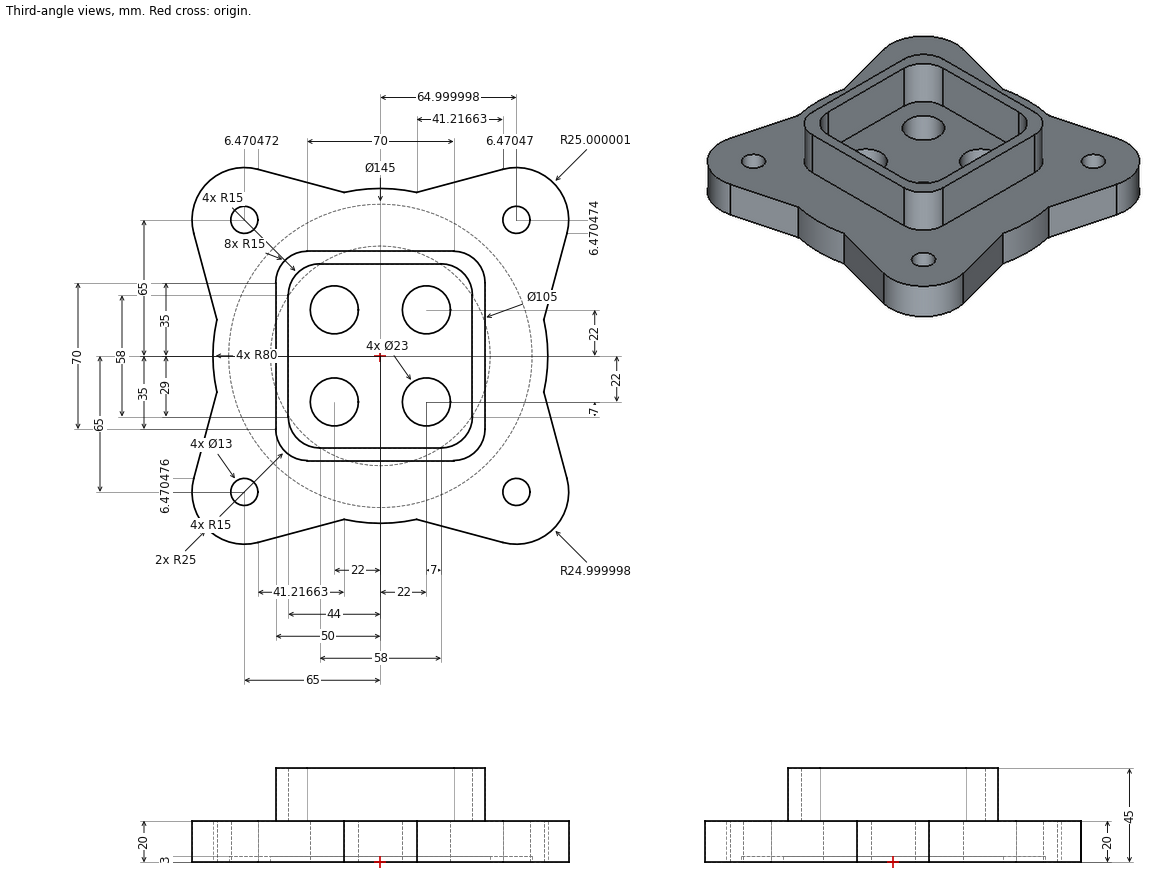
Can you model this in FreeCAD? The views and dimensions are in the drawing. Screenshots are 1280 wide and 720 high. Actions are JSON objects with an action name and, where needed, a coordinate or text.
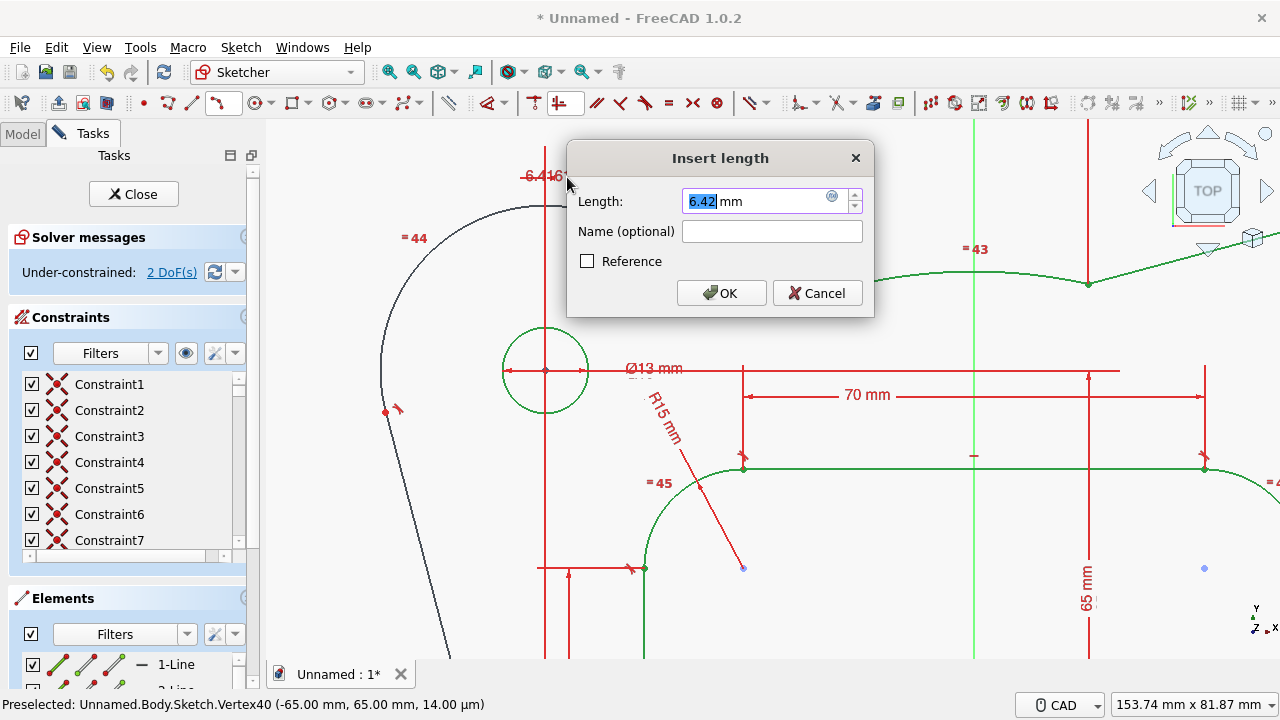
{"action": "type", "text": "6.470472"}
{"action": "key", "text": "Return"}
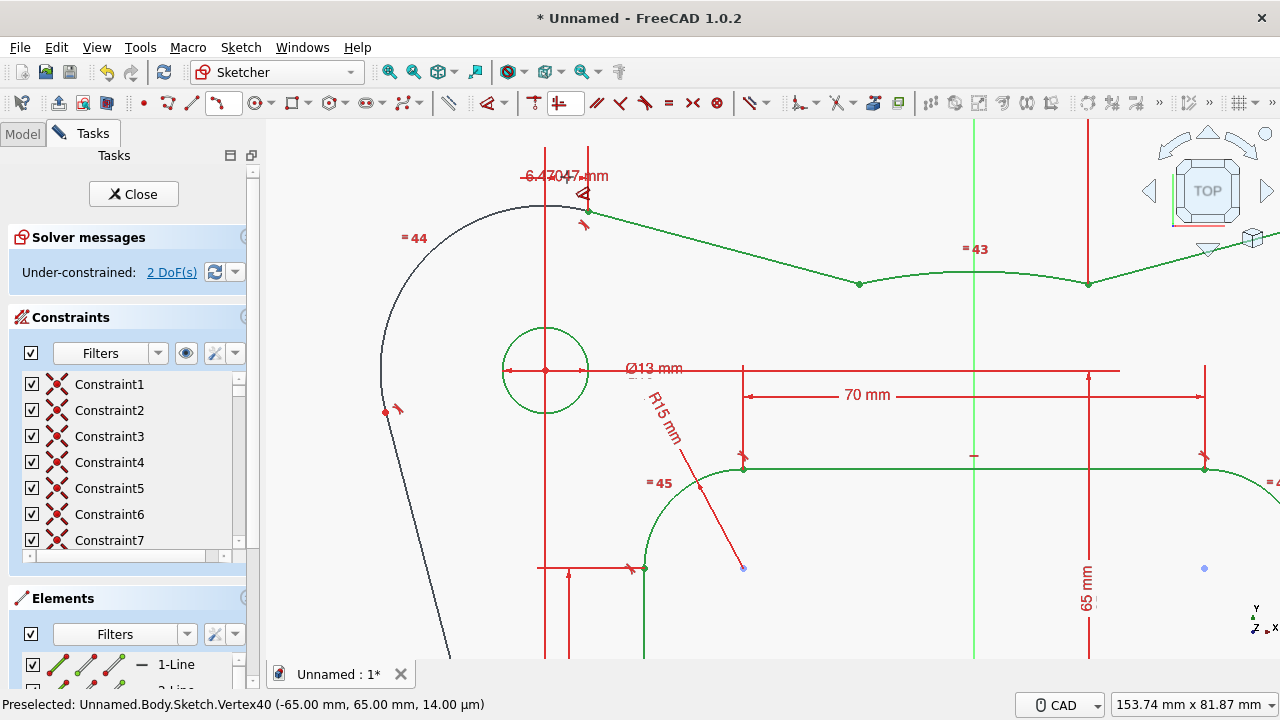
{"action": "left_click", "coordinate": [386, 412]}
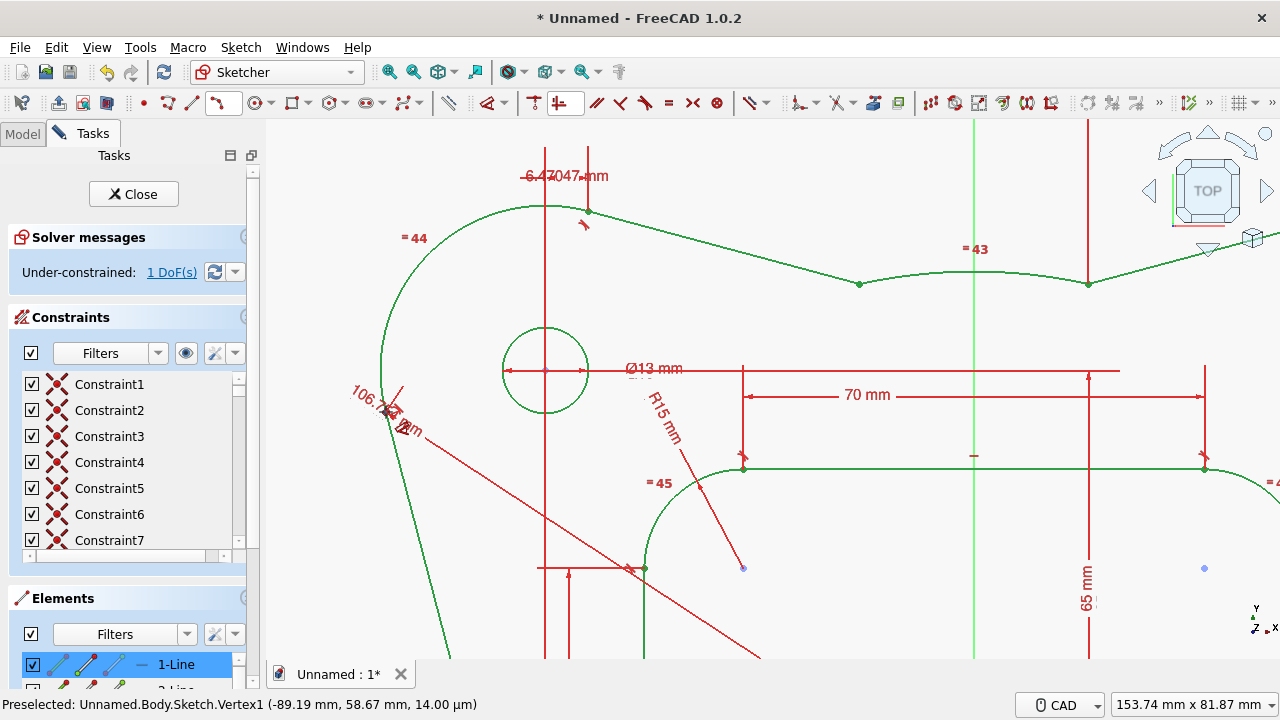
{"action": "left_click", "coordinate": [545, 371]}
{"action": "left_click", "coordinate": [352, 391]}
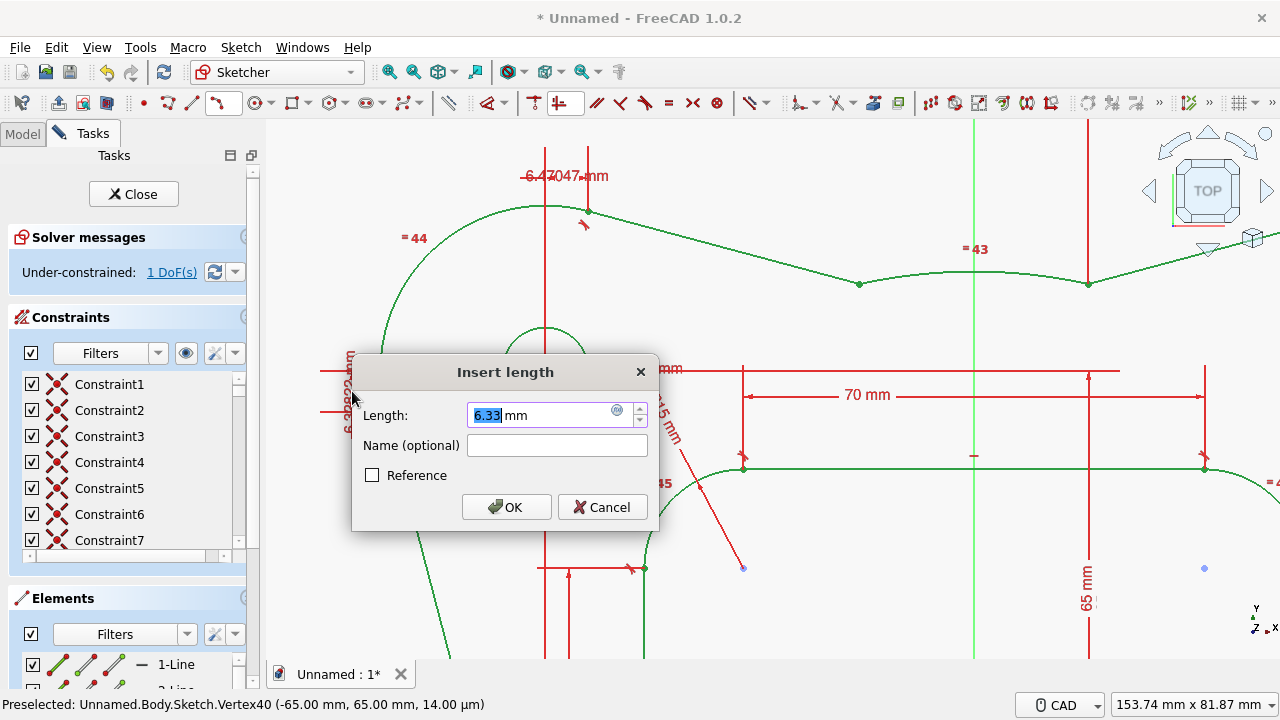
{"action": "type", "text": "6.470476"}
{"action": "key", "text": "Return"}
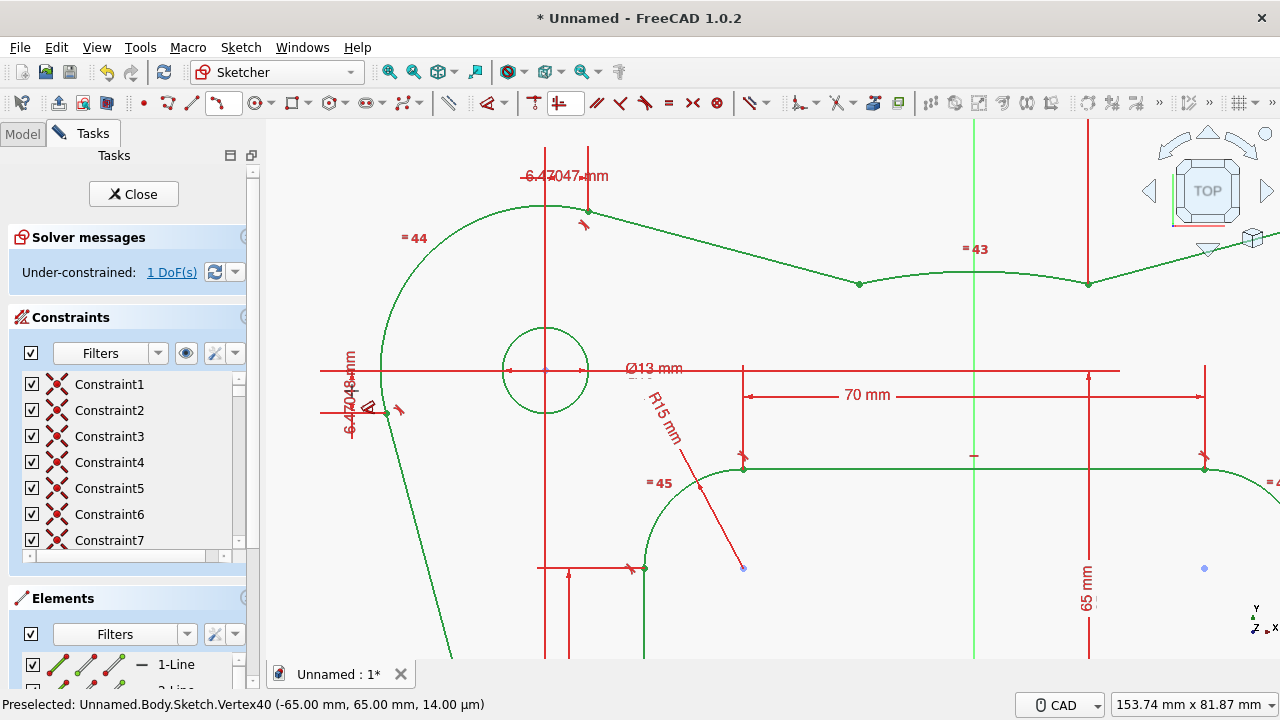
{"action": "scroll", "coordinate": [588, 212], "scroll_direction": "down", "scroll_amount": 6}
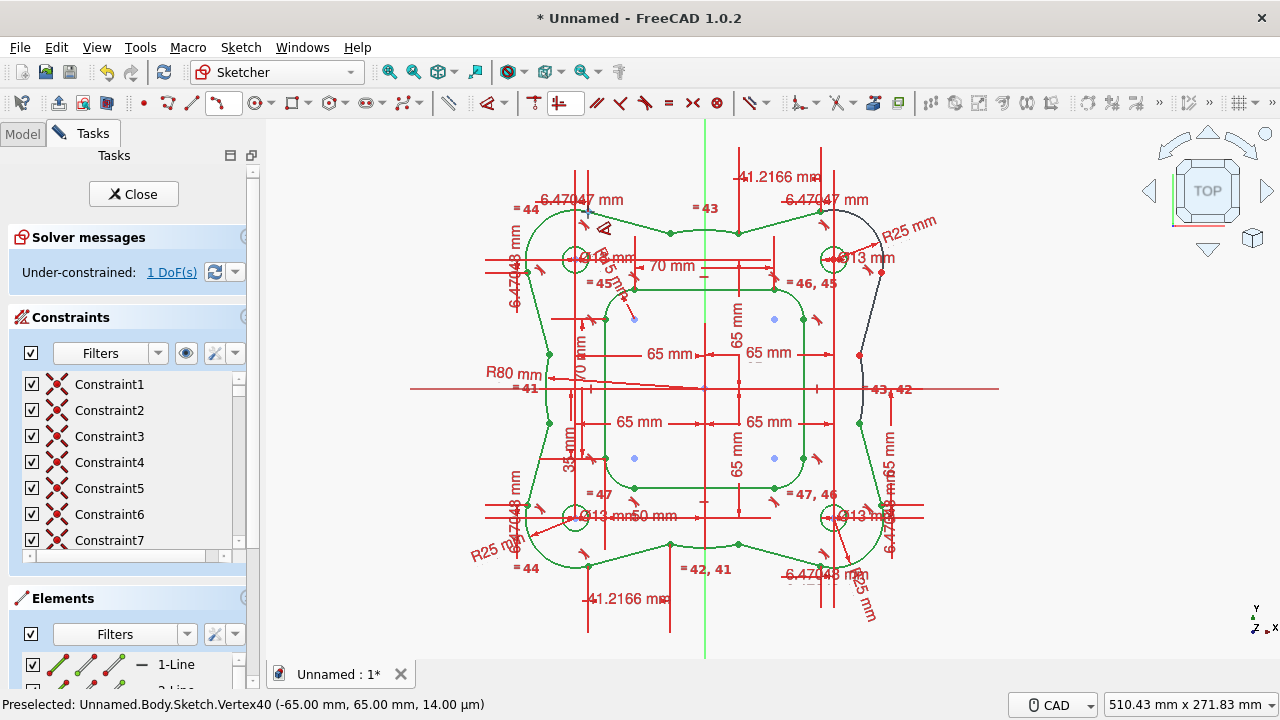
{"action": "scroll", "coordinate": [882, 272], "scroll_direction": "up", "scroll_amount": 6}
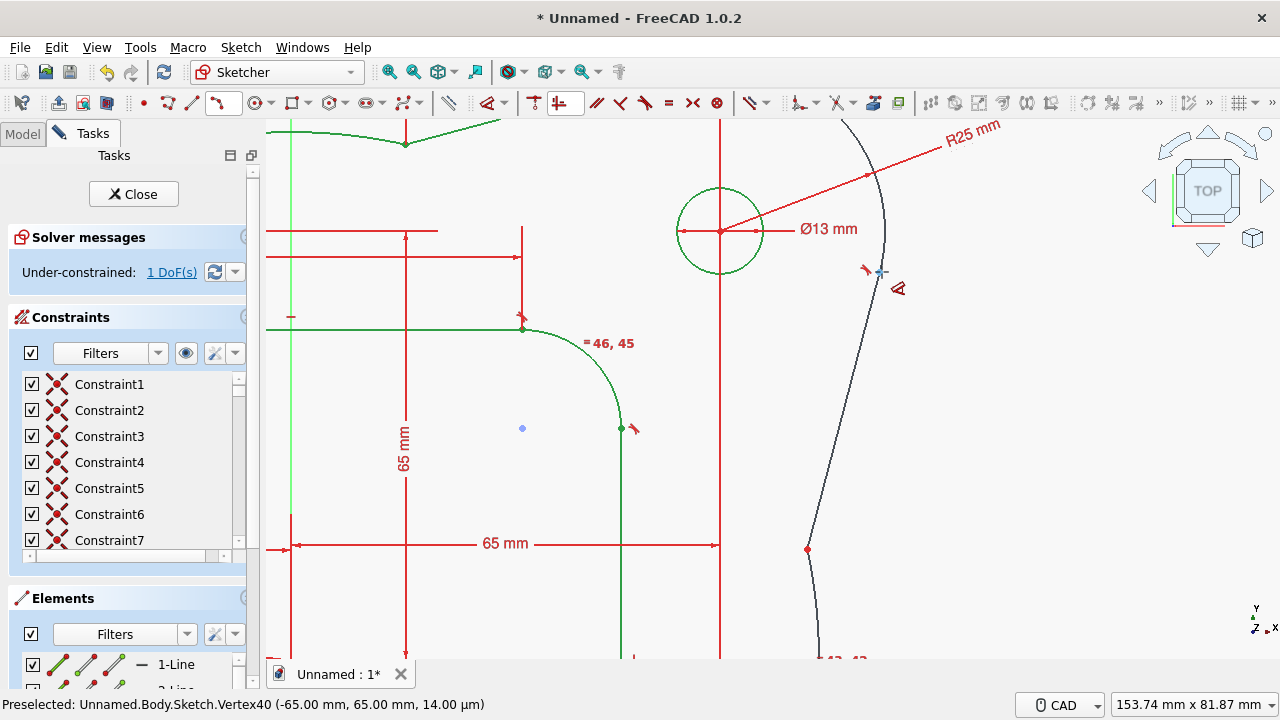
{"action": "left_click", "coordinate": [880, 273]}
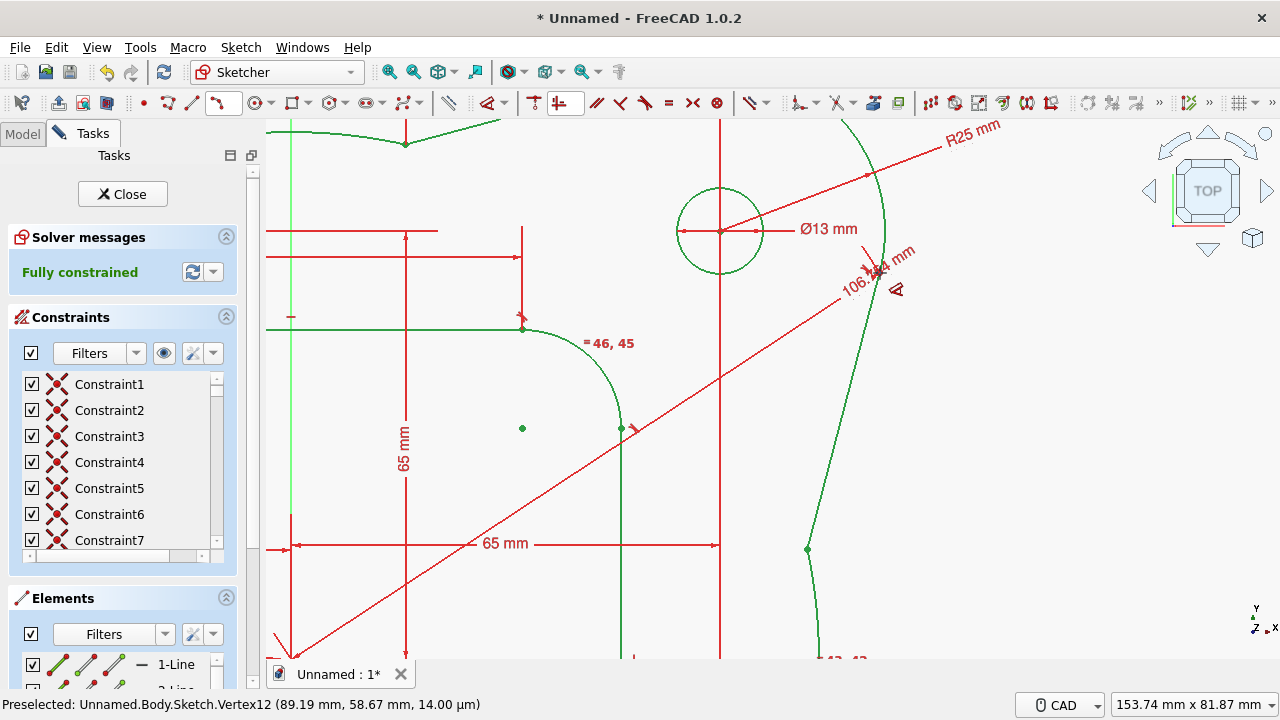
{"action": "left_click", "coordinate": [720, 231]}
{"action": "left_click", "coordinate": [914, 252]}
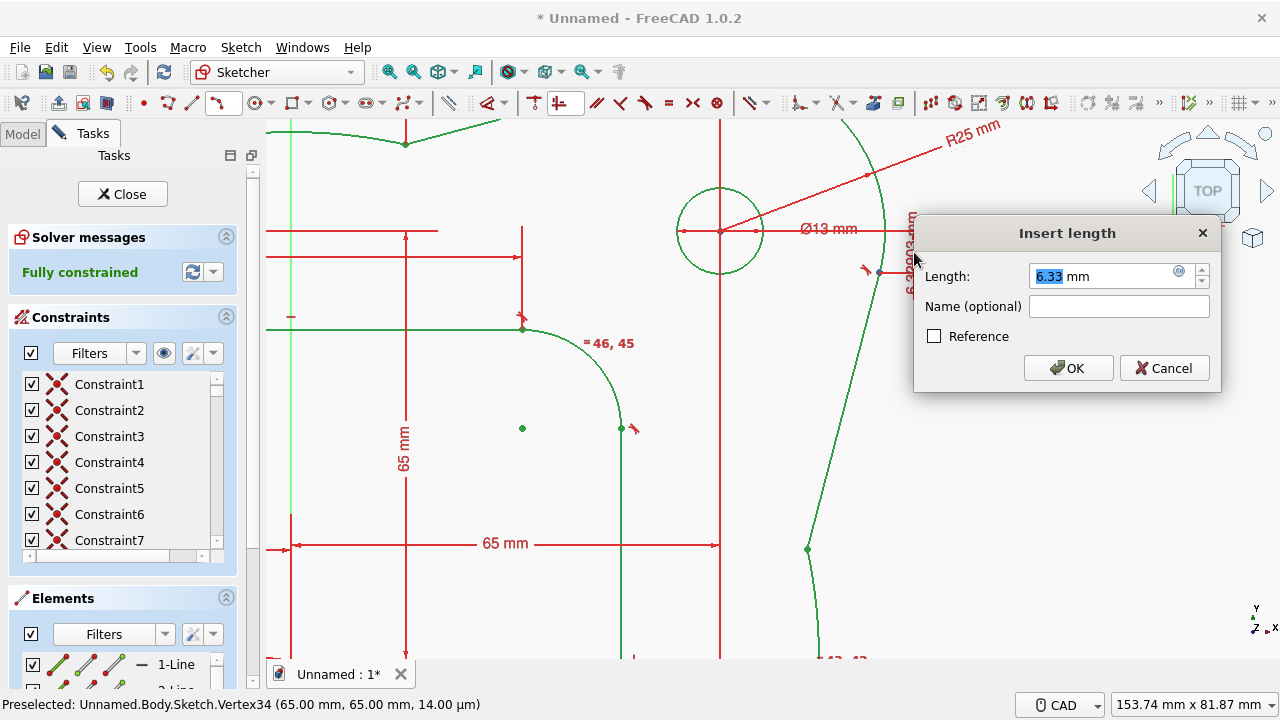
{"action": "type", "text": "6.470474"}
{"action": "key", "text": "Return"}
{"action": "key", "text": "Escape"}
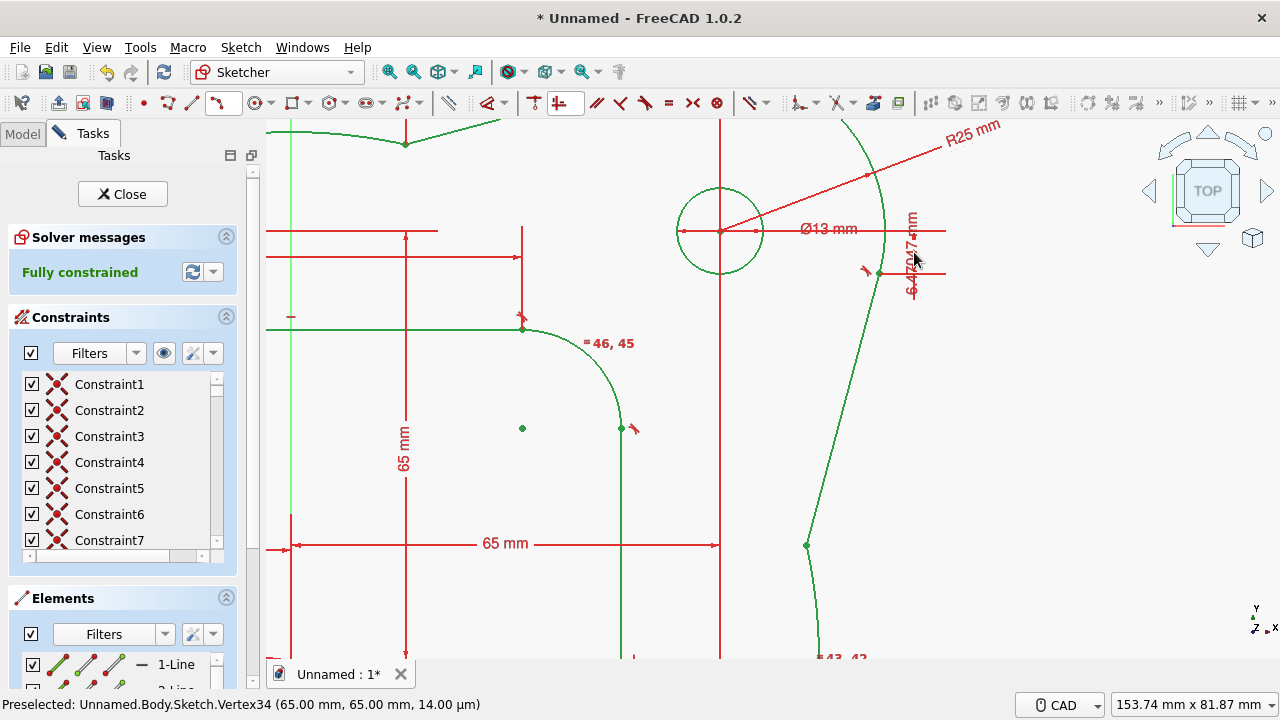
{"action": "left_click", "coordinate": [123, 194]}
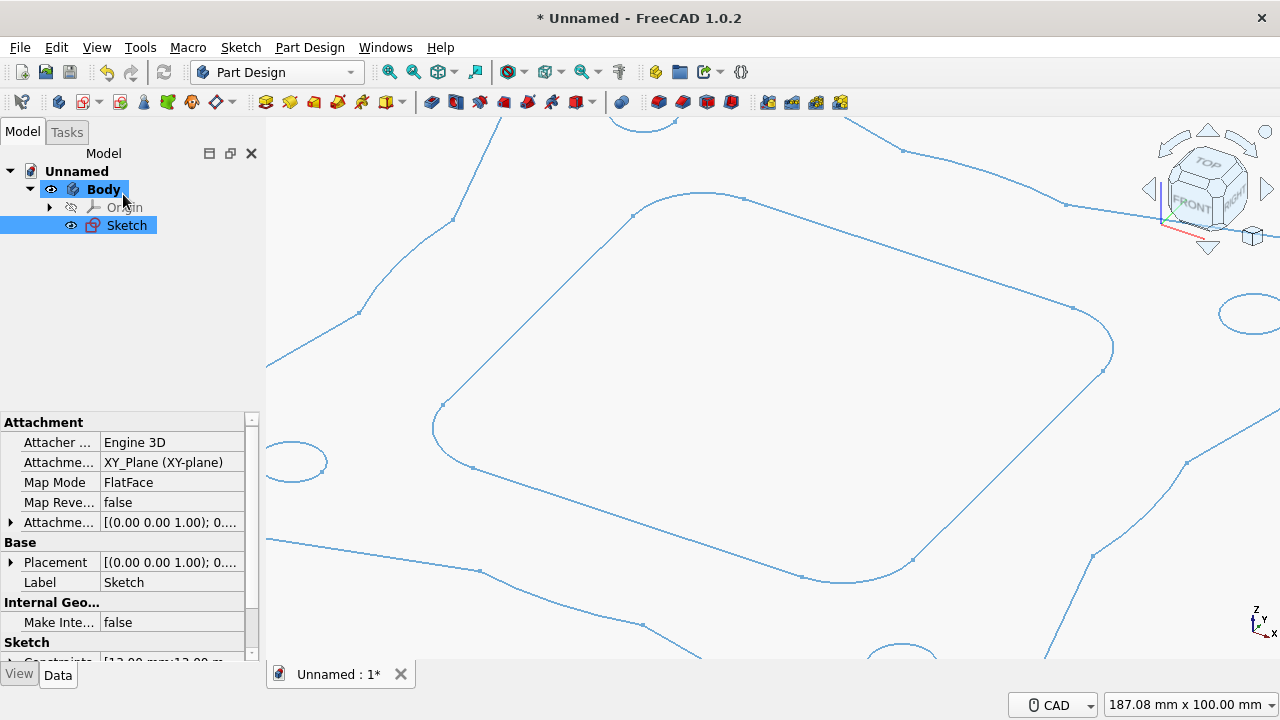
{"action": "left_click", "coordinate": [266, 102]}